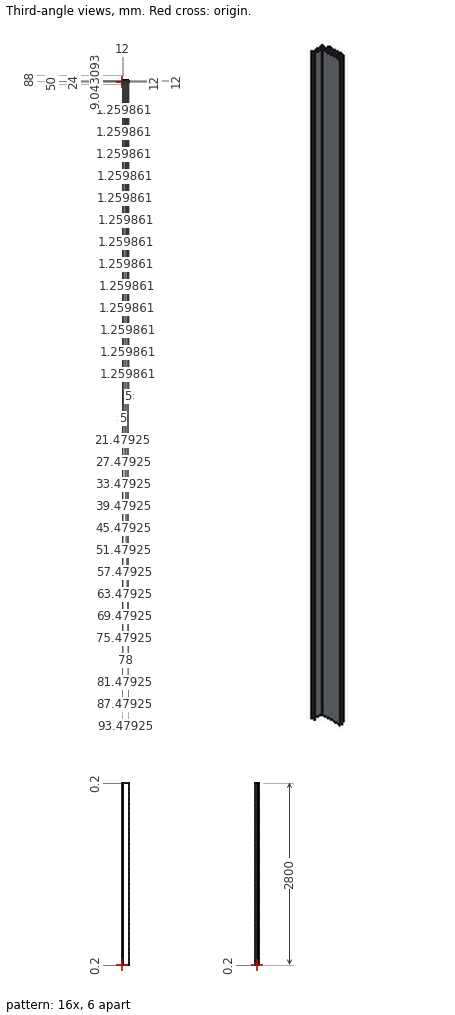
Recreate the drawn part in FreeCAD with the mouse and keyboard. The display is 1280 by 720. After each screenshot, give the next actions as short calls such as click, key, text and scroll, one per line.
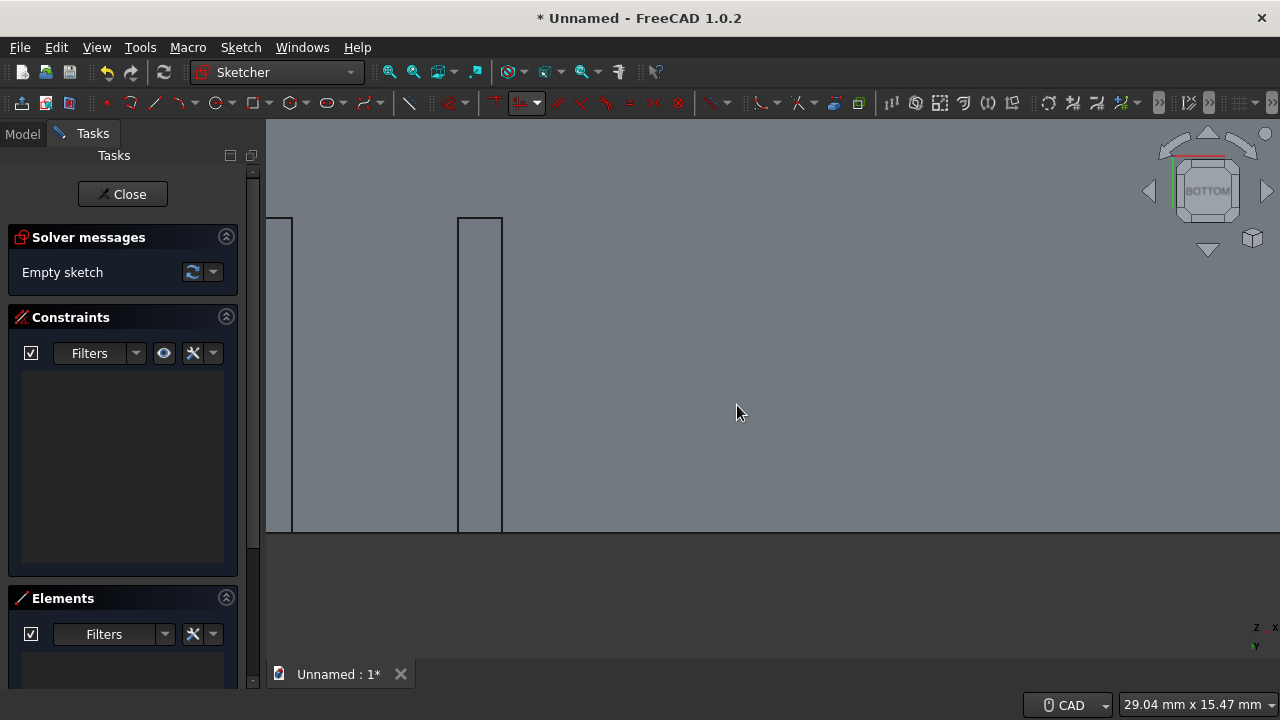
click(254, 104)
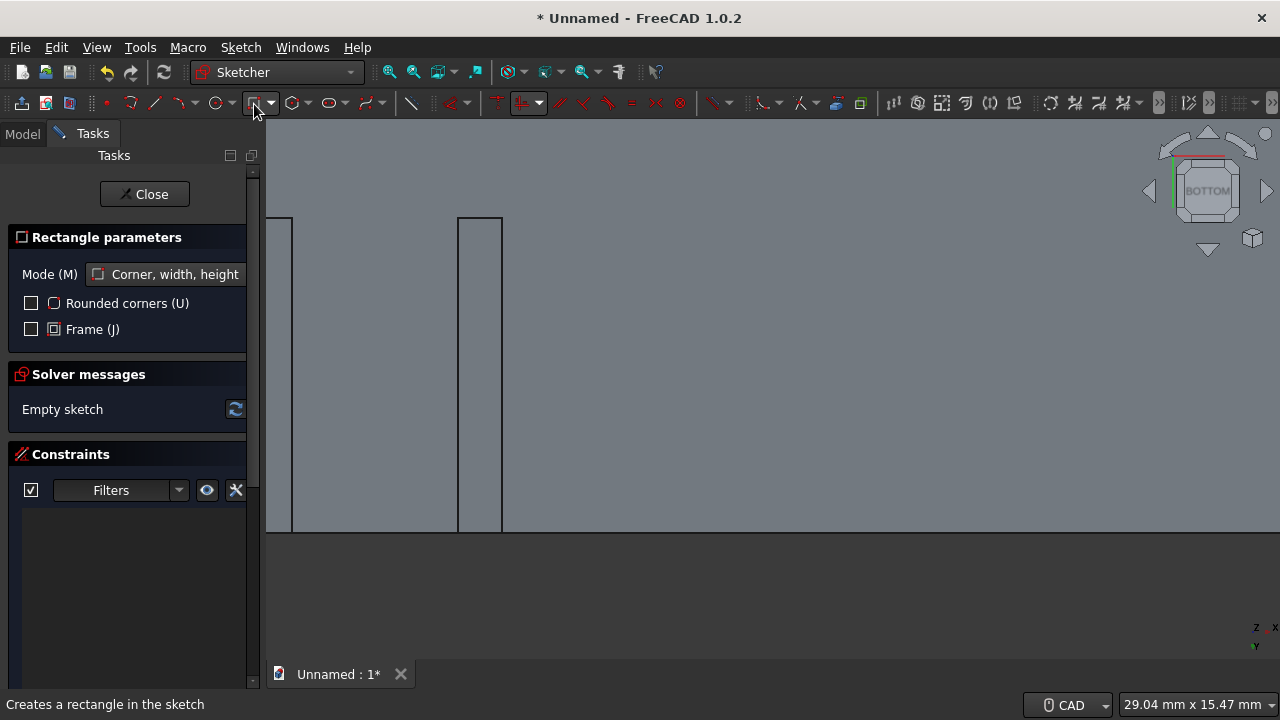
click(667, 218)
move(711, 533)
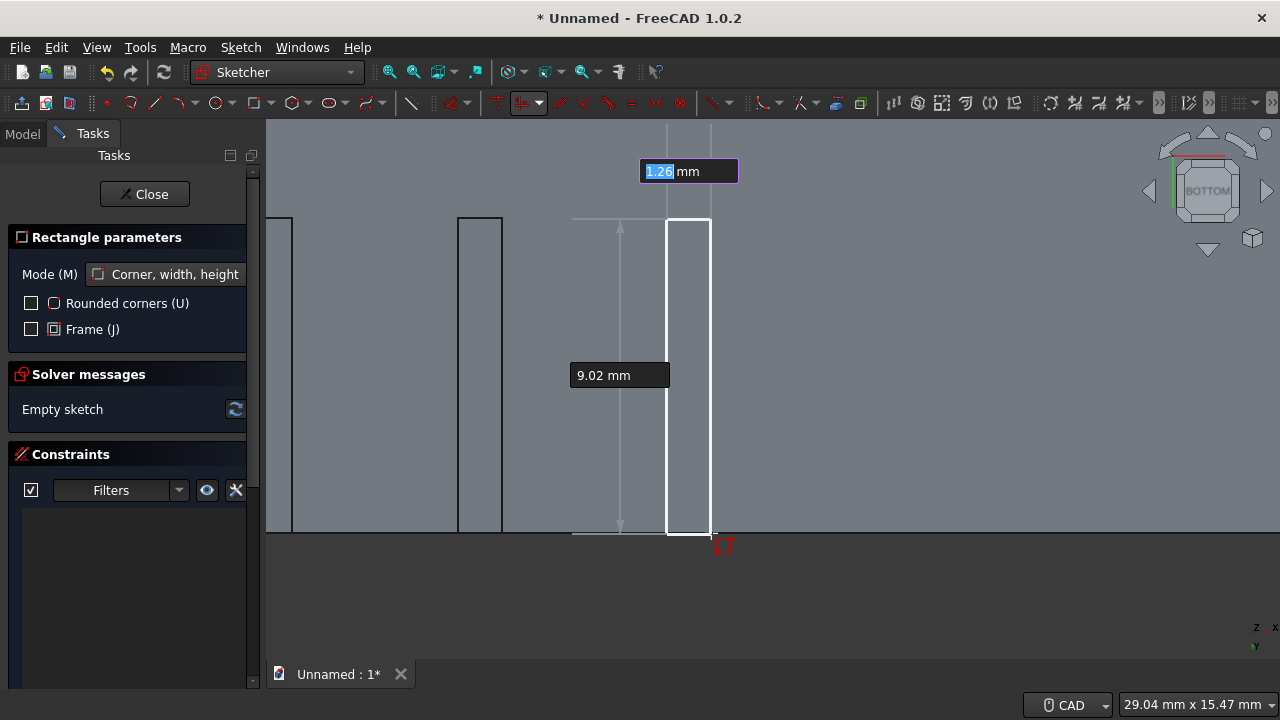
text(1.259861)
key(Tab)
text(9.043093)
key(Return)
key(Escape)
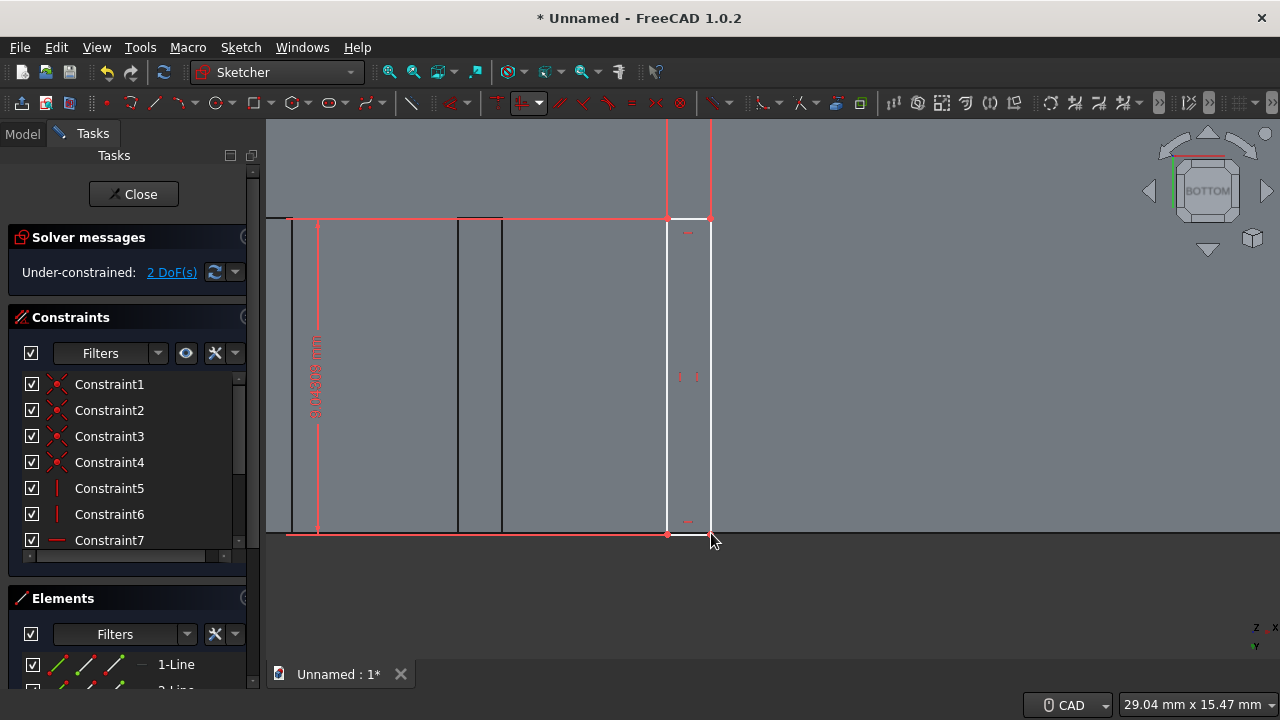
click(450, 104)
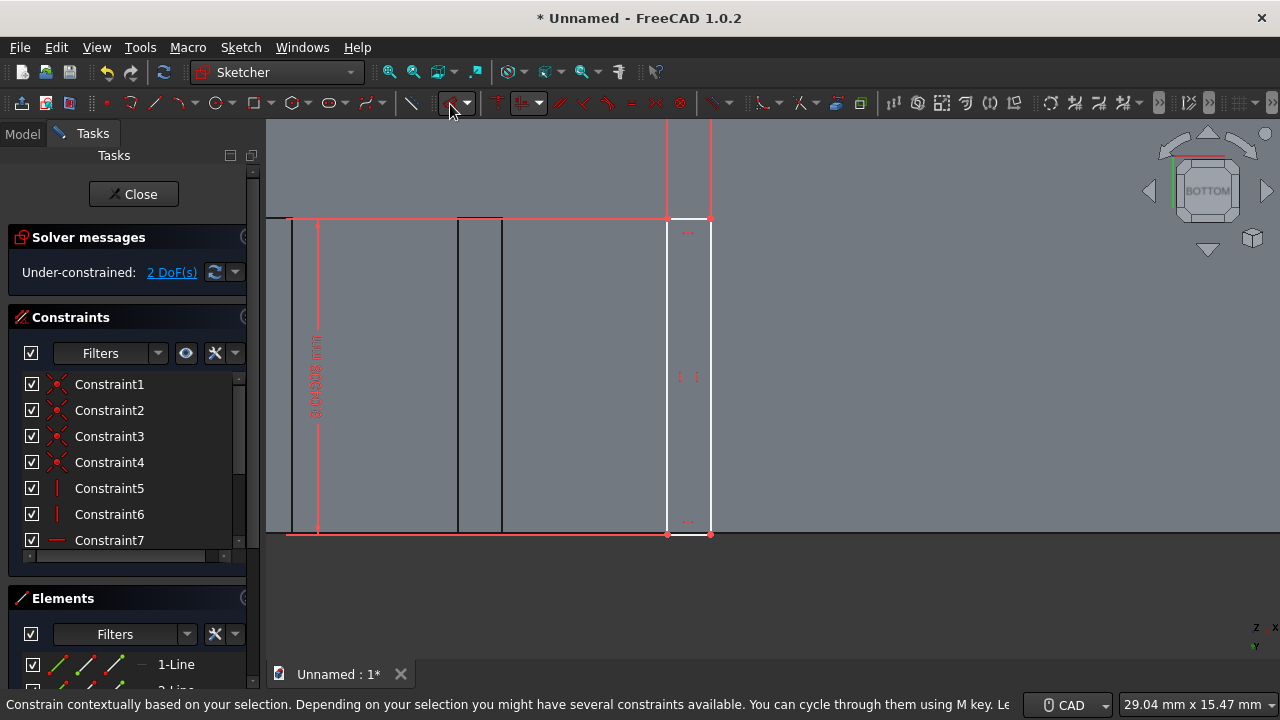
click(667, 535)
click(701, 205)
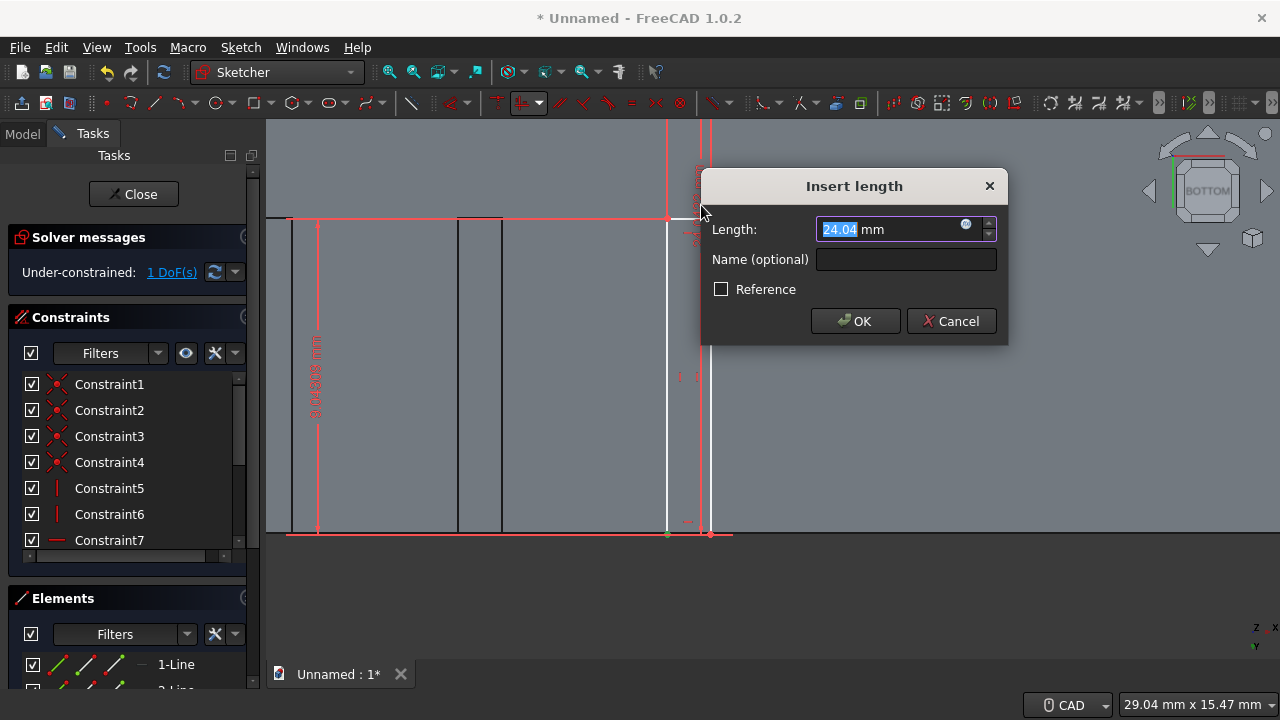
text(24)
key(Return)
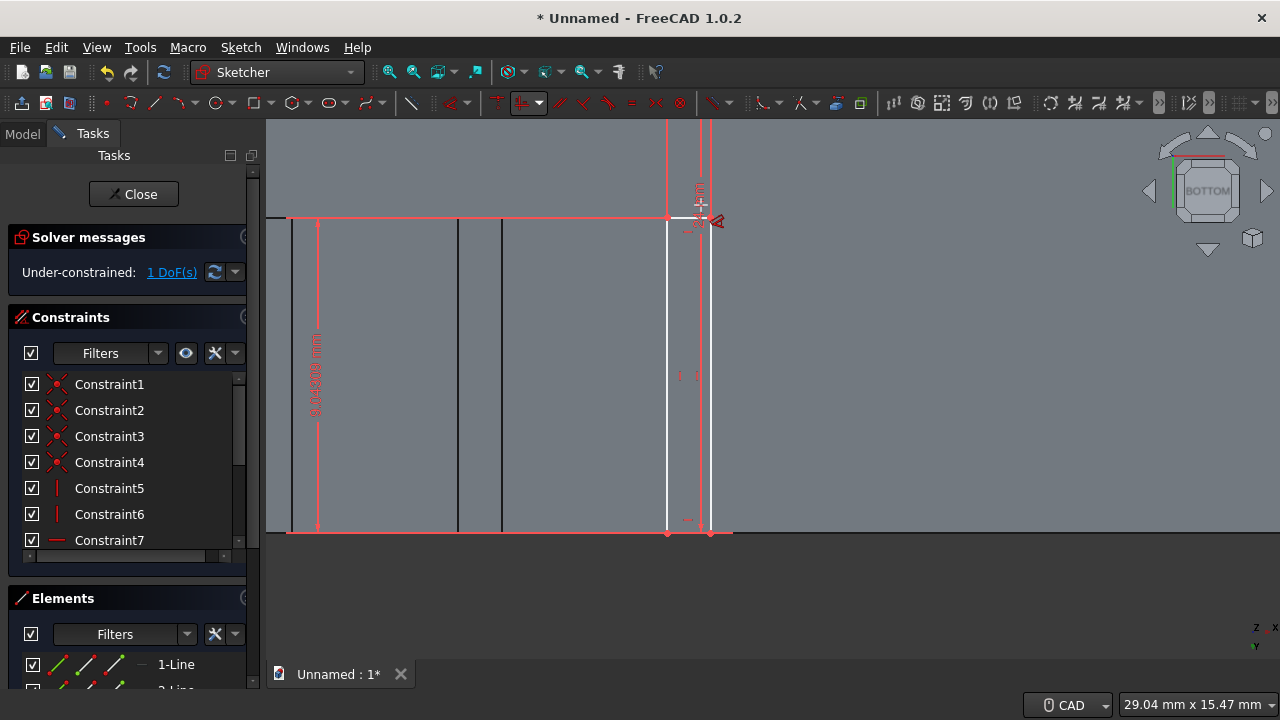
click(667, 218)
click(480, 252)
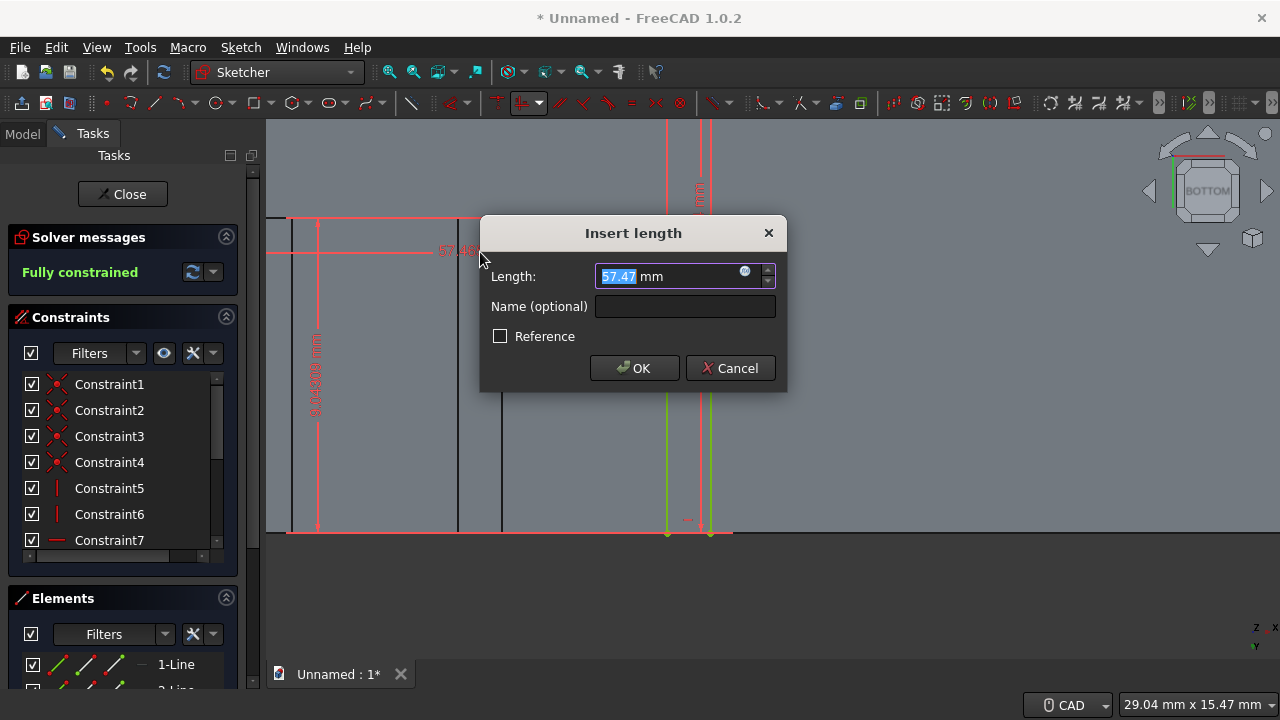
text(57.47925)
key(Return)
key(Escape)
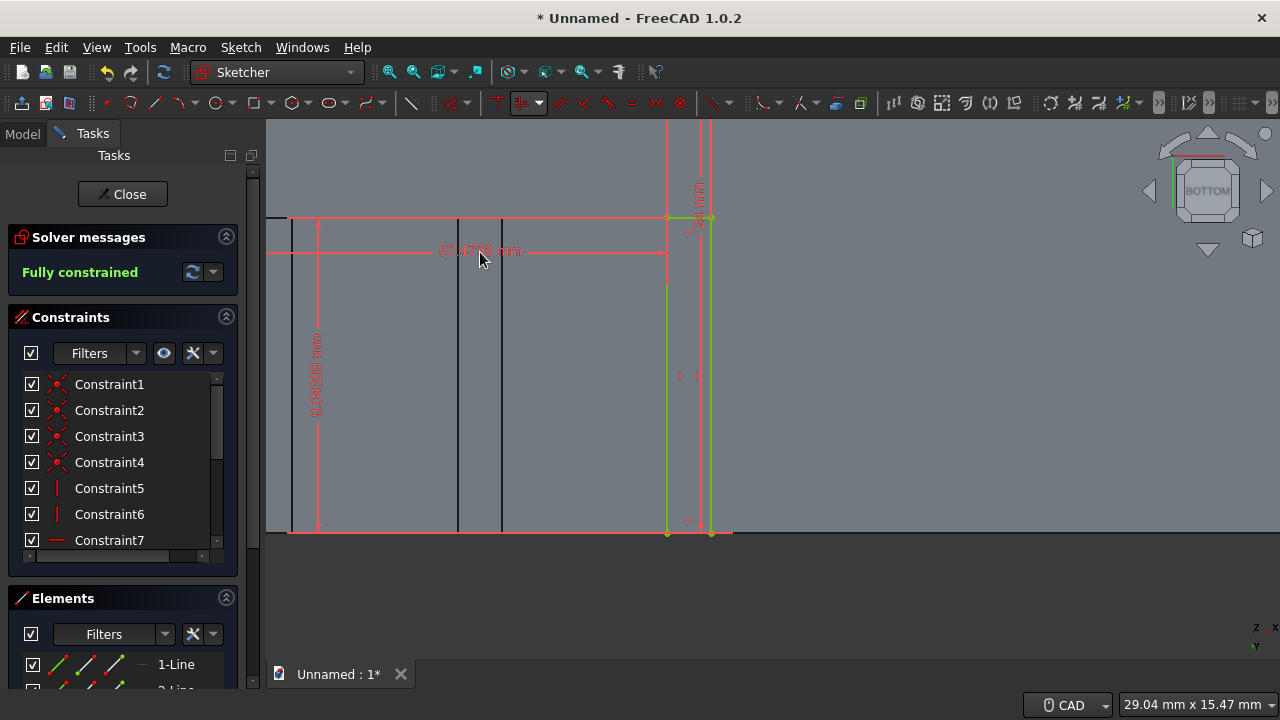
click(123, 194)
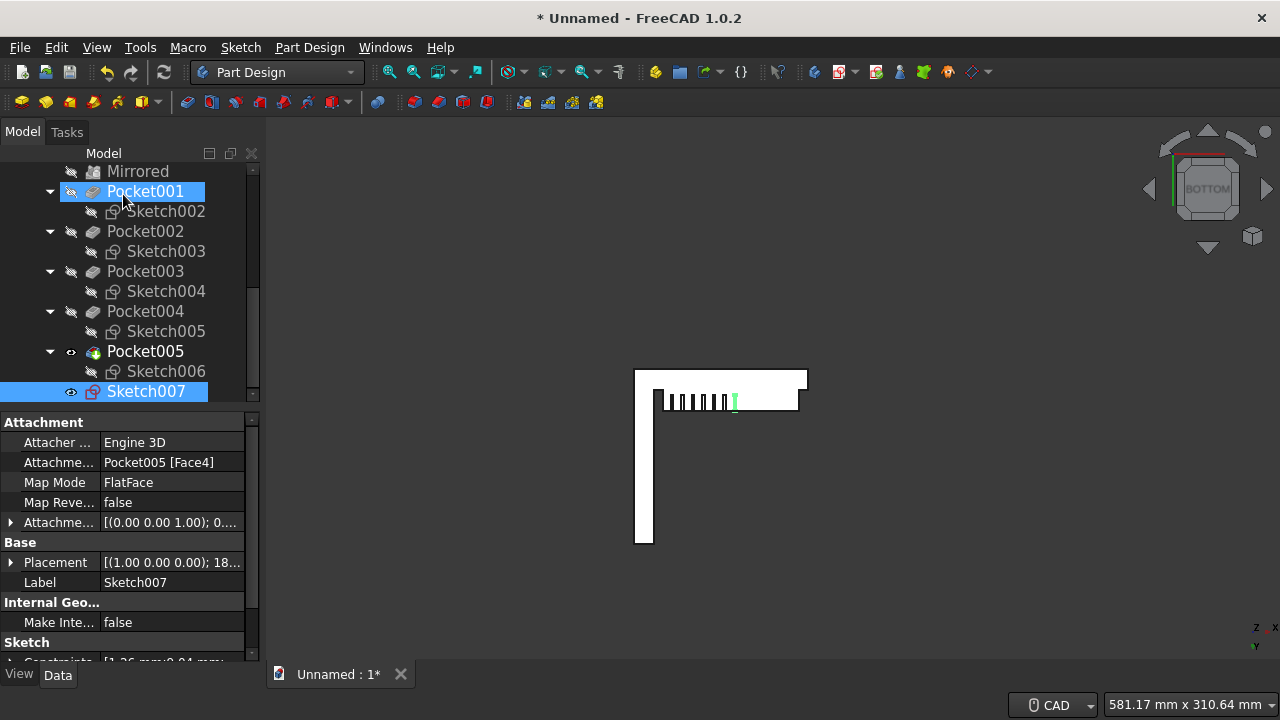
click(188, 102)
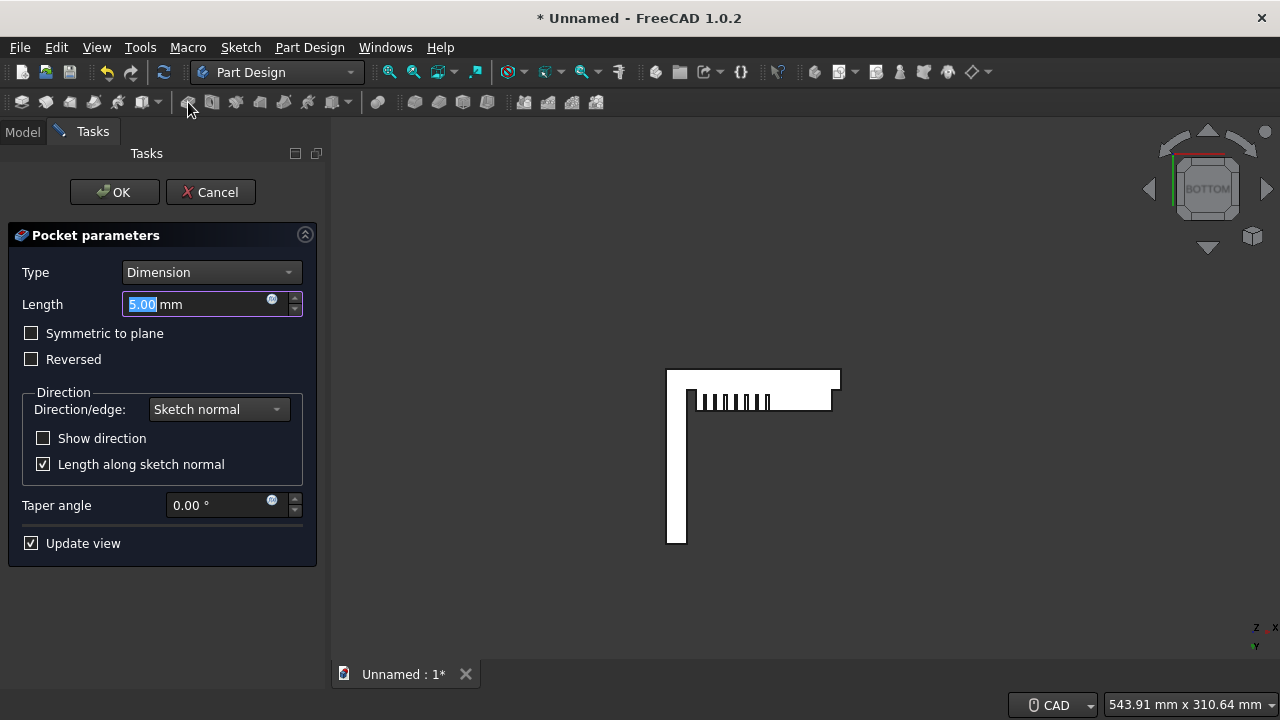
text(0.2)
key(Tab)